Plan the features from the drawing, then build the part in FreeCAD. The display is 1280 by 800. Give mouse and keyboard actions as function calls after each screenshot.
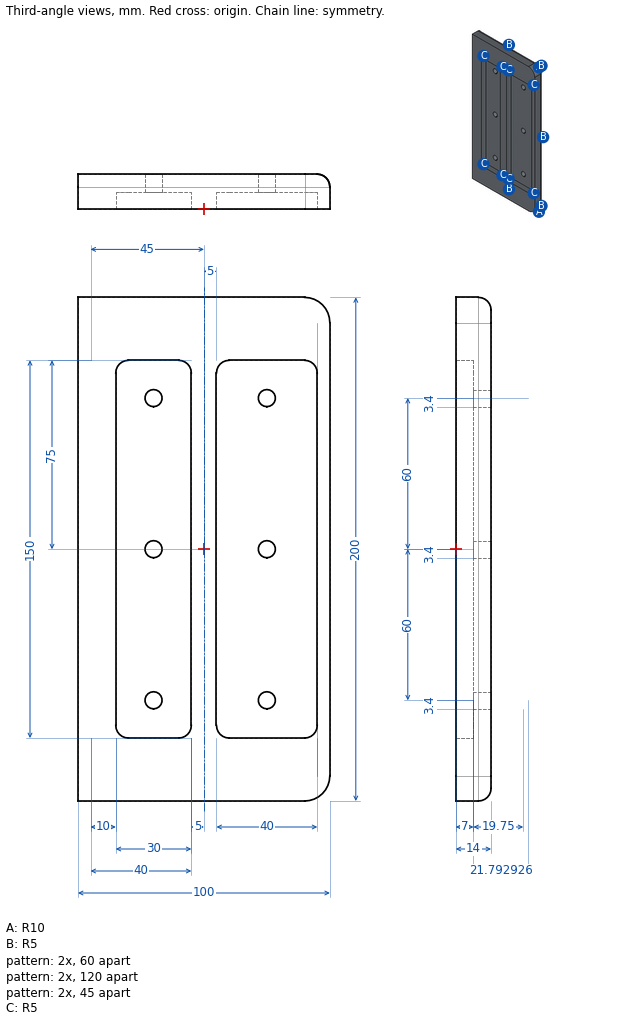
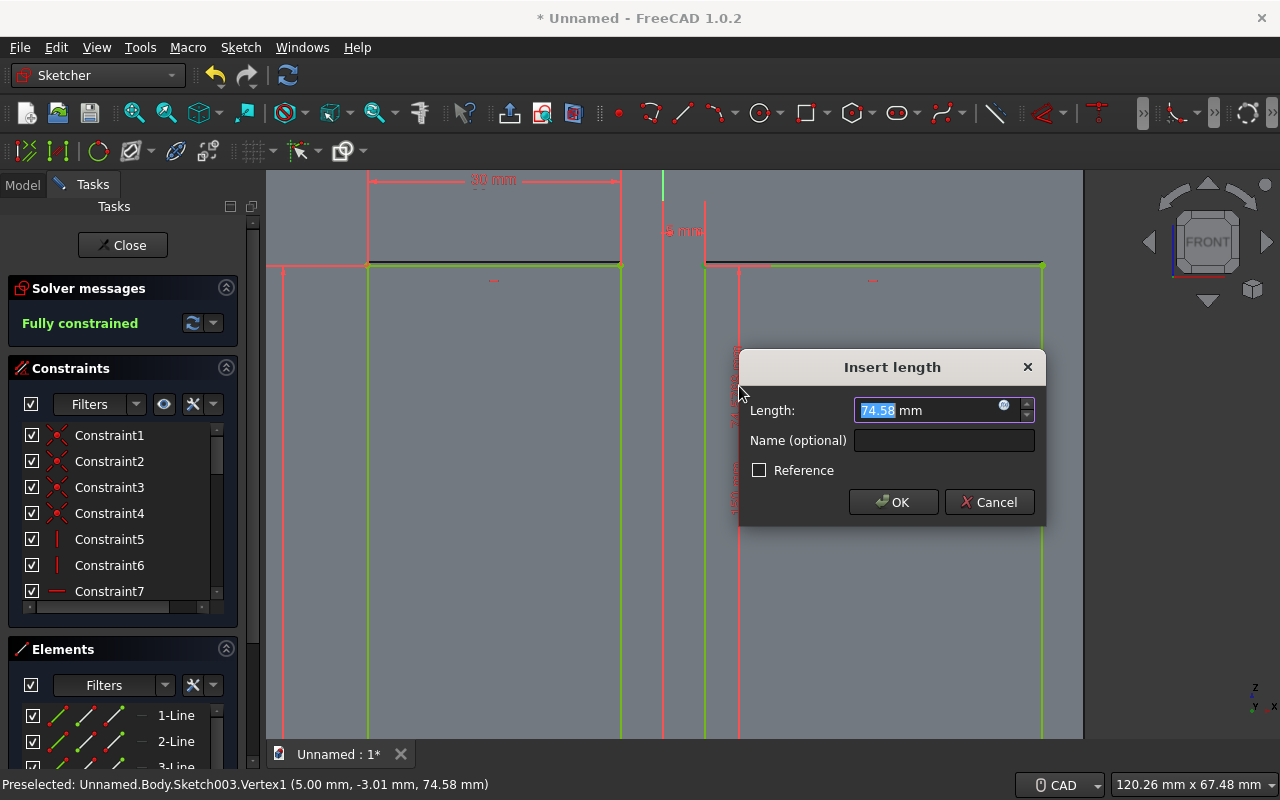
text(75)
key(Return)
key(Escape)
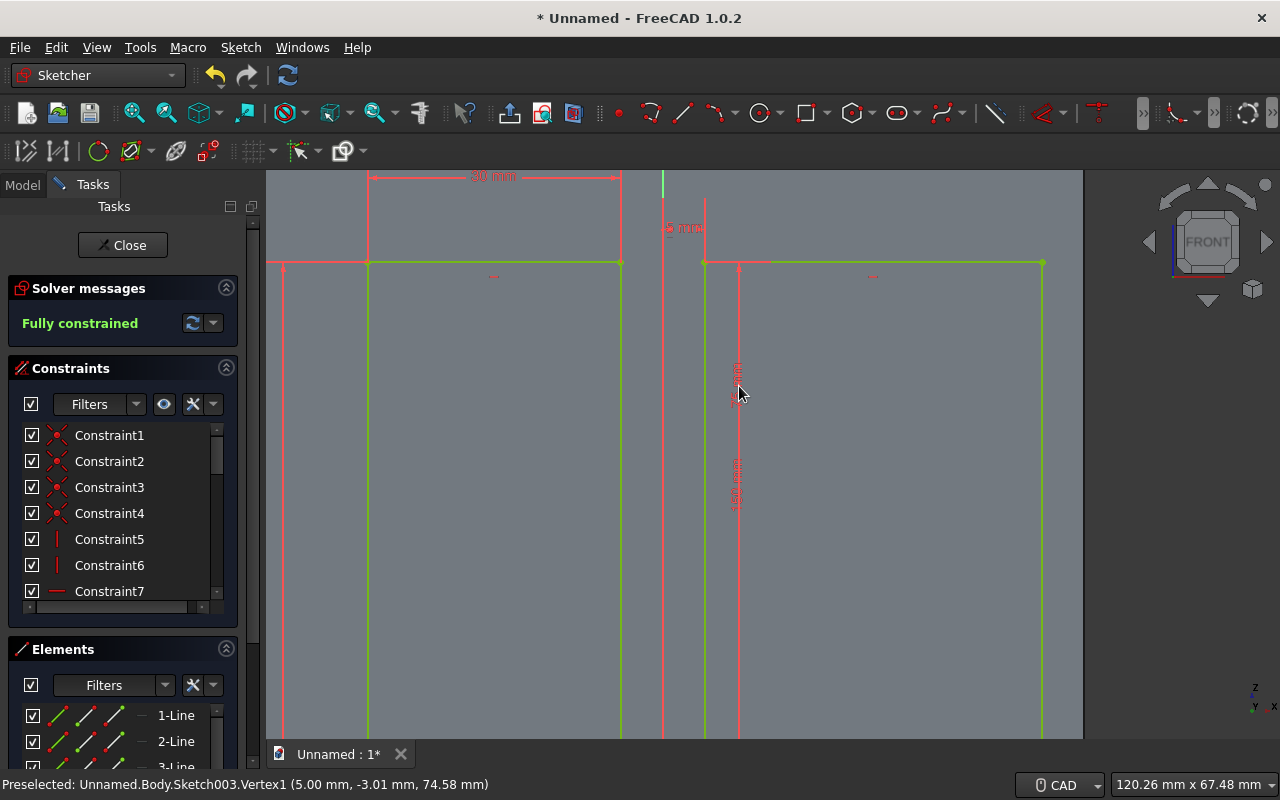
click(123, 245)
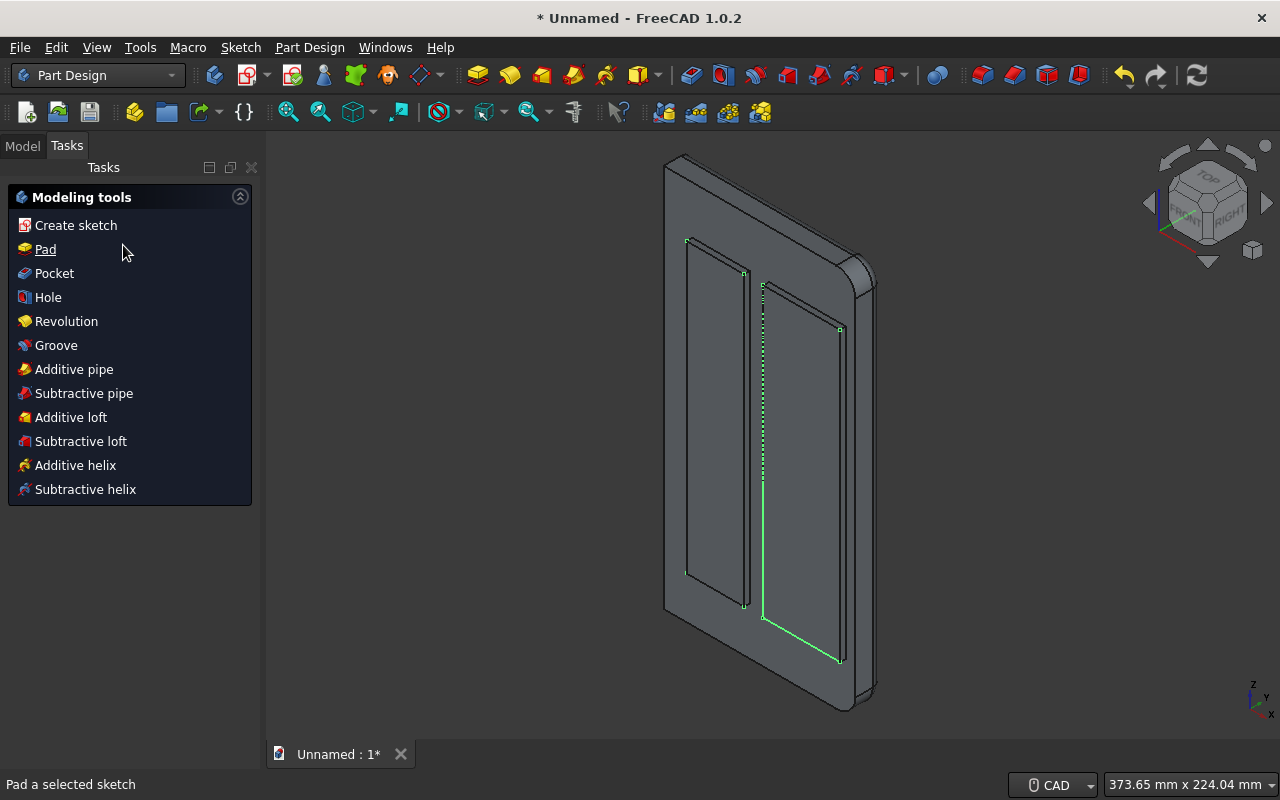
click(692, 76)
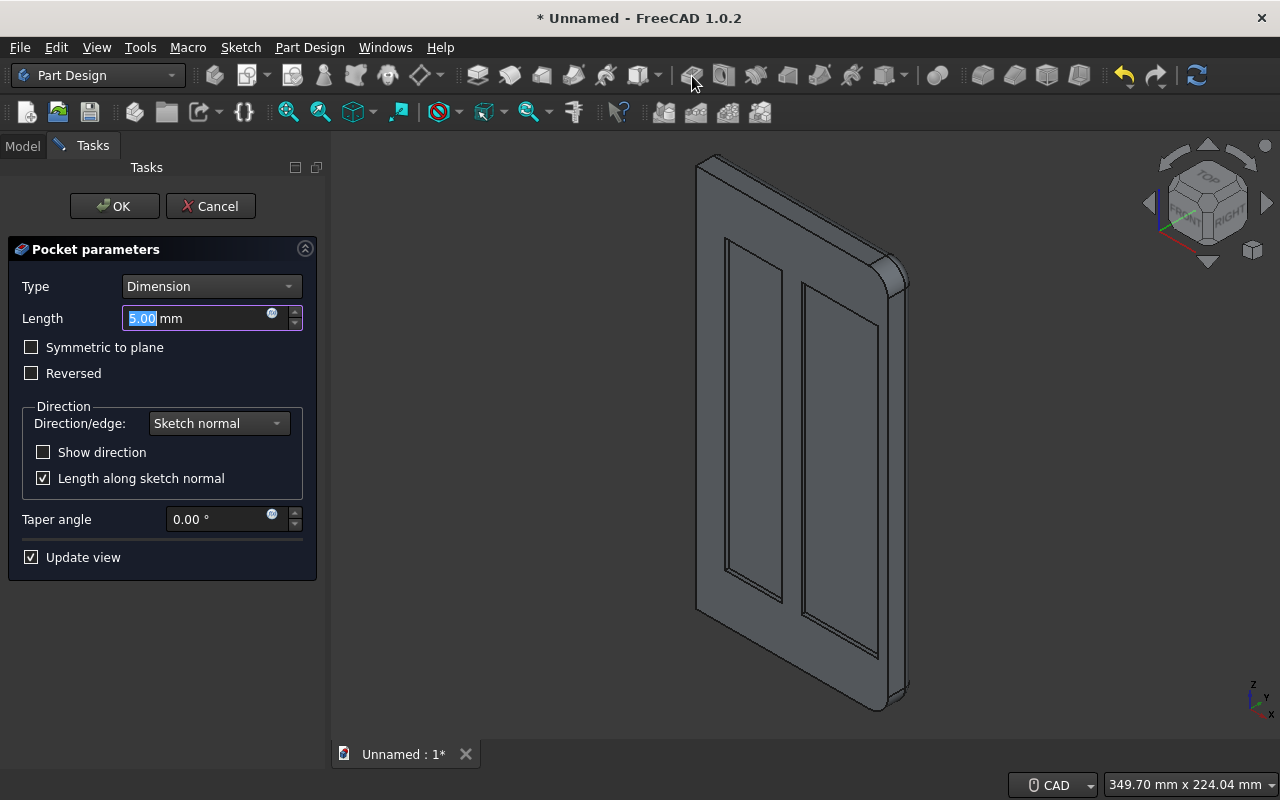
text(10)
key(Tab)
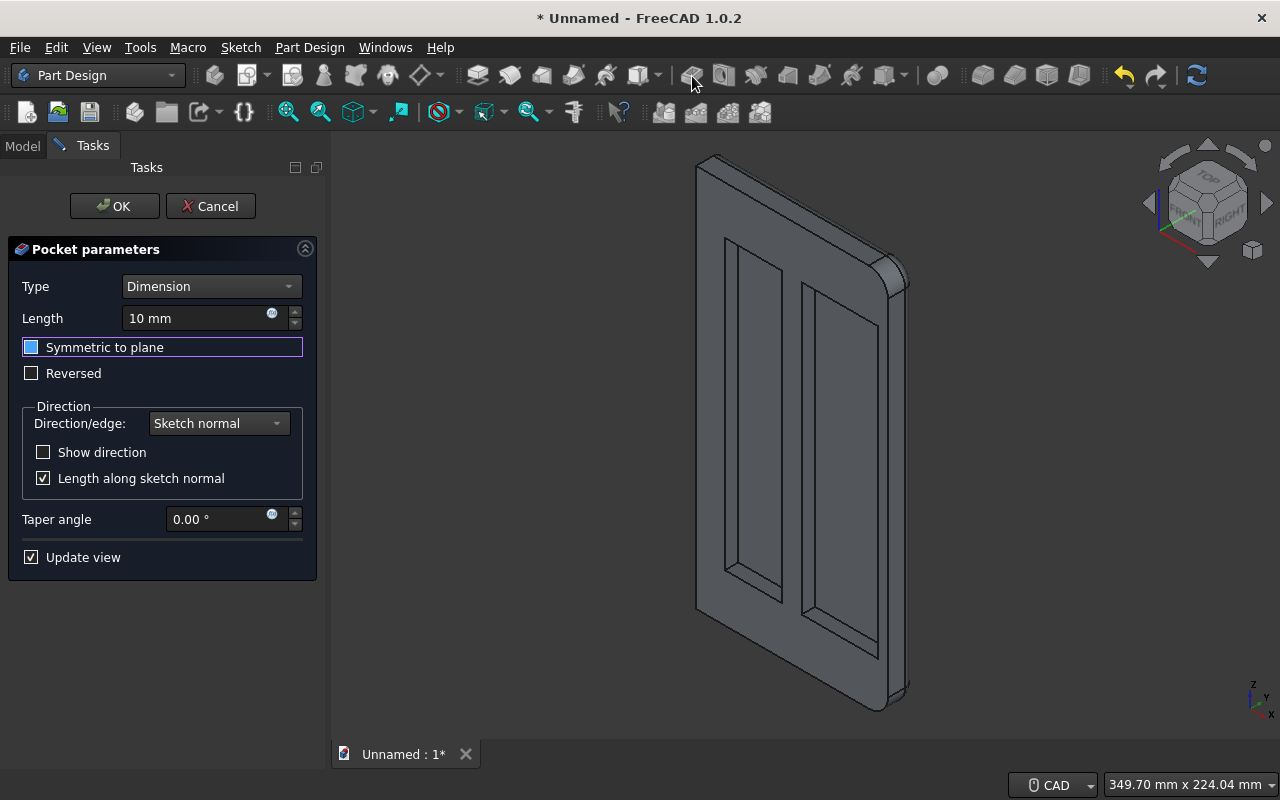
click(115, 206)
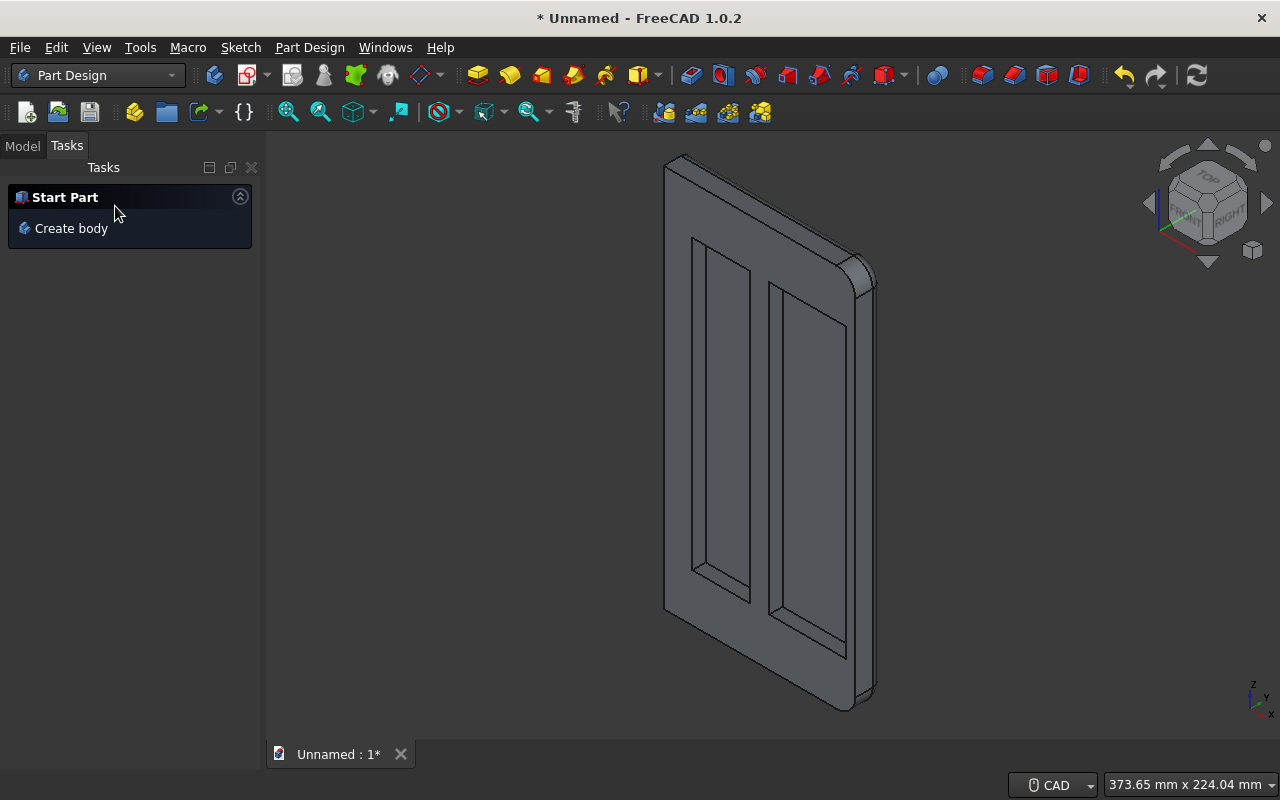
click(23, 145)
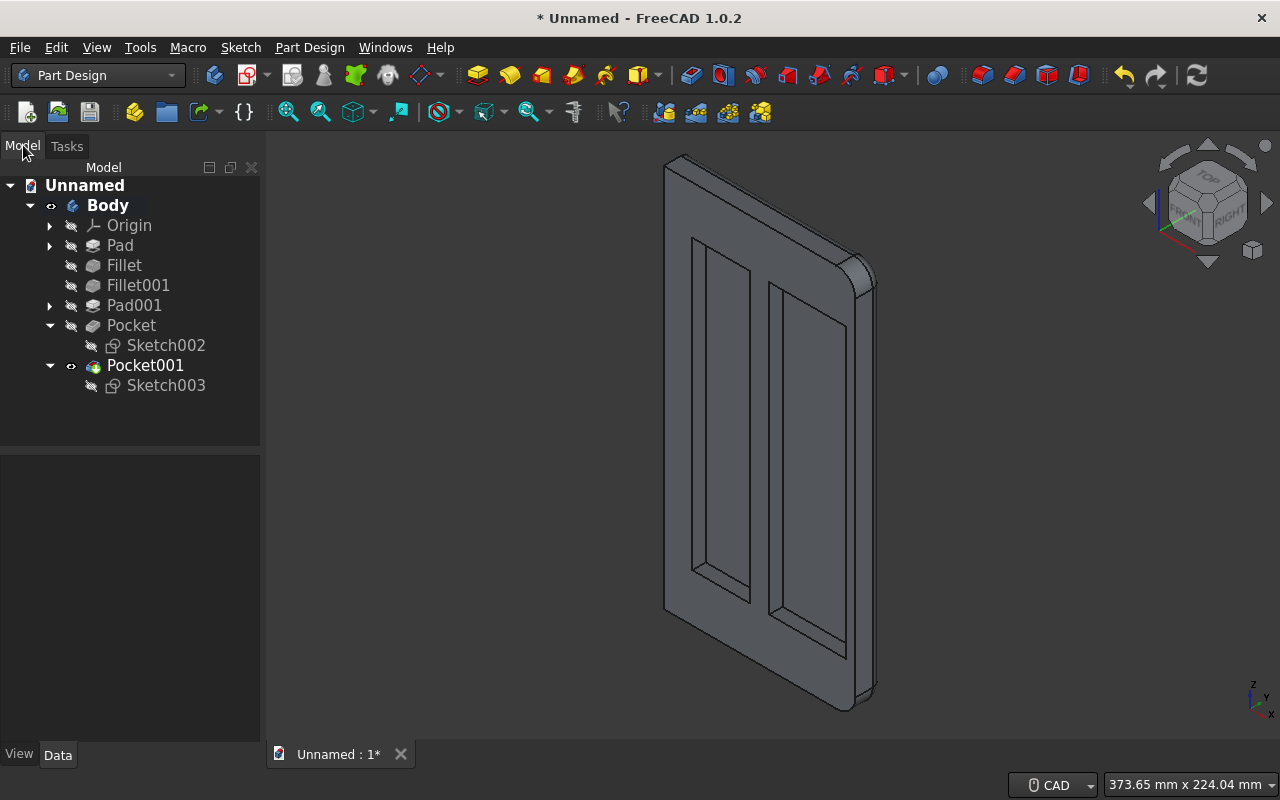
click(50, 226)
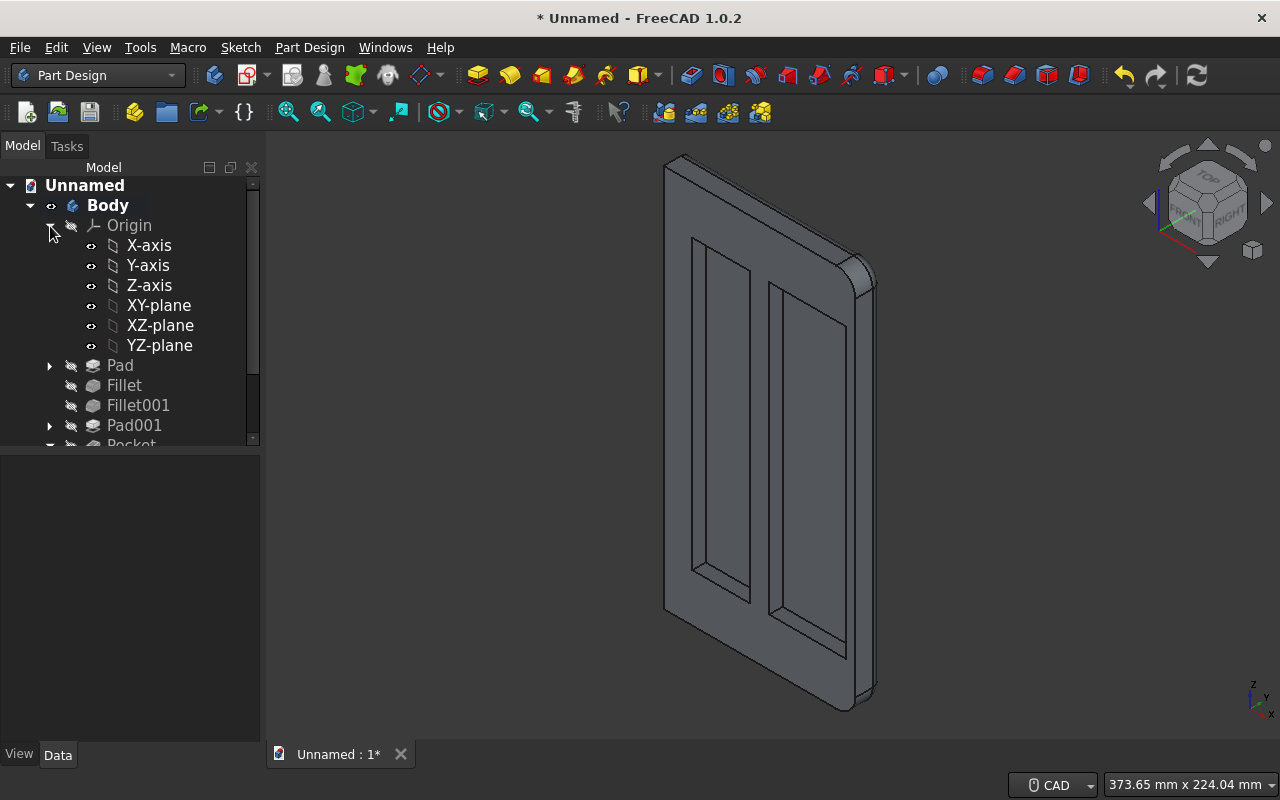
click(136, 346)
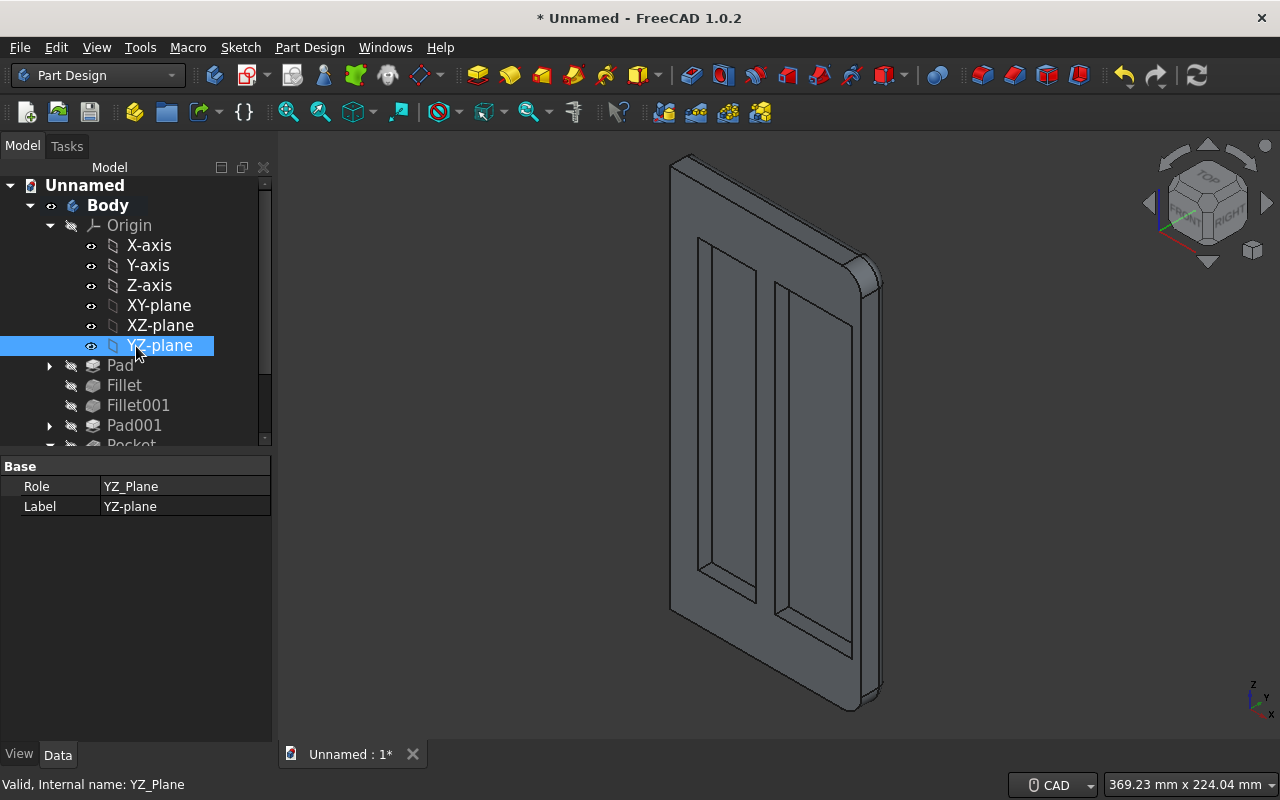
click(420, 76)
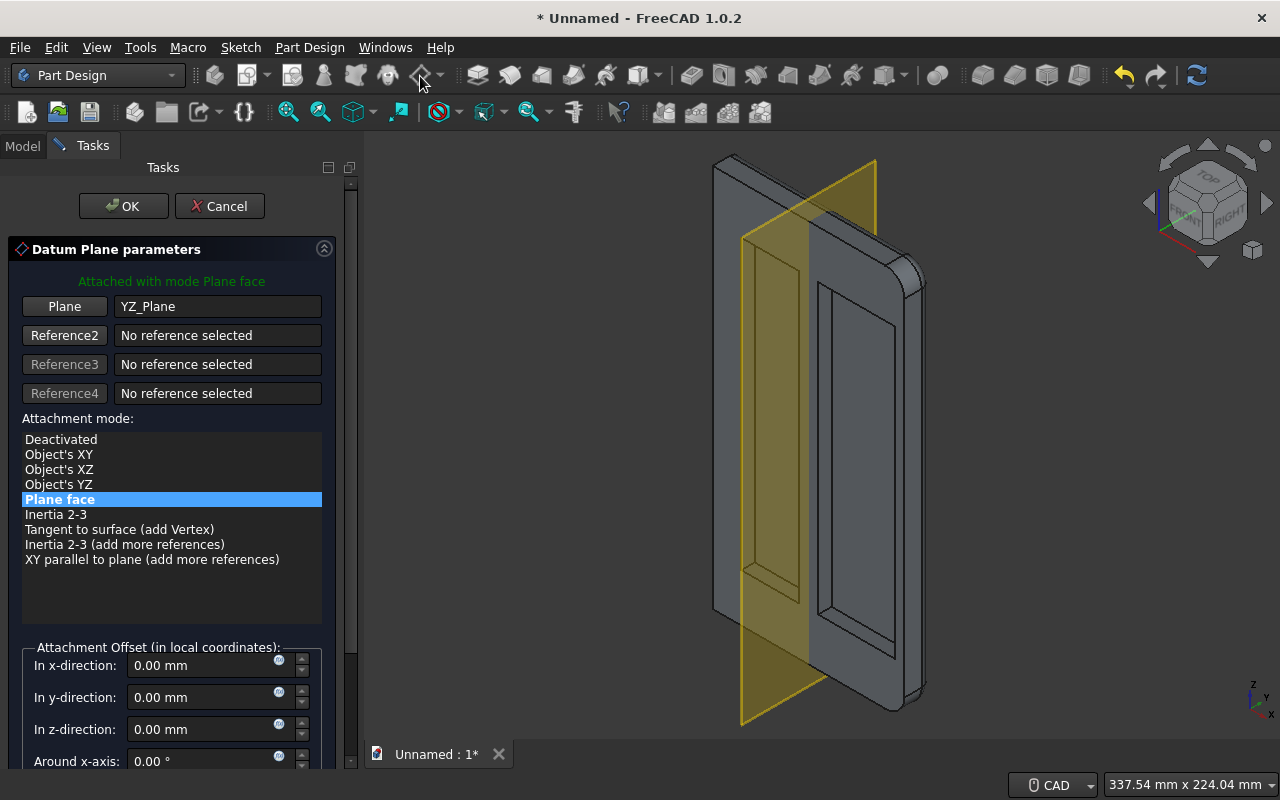
triple_click(210, 729)